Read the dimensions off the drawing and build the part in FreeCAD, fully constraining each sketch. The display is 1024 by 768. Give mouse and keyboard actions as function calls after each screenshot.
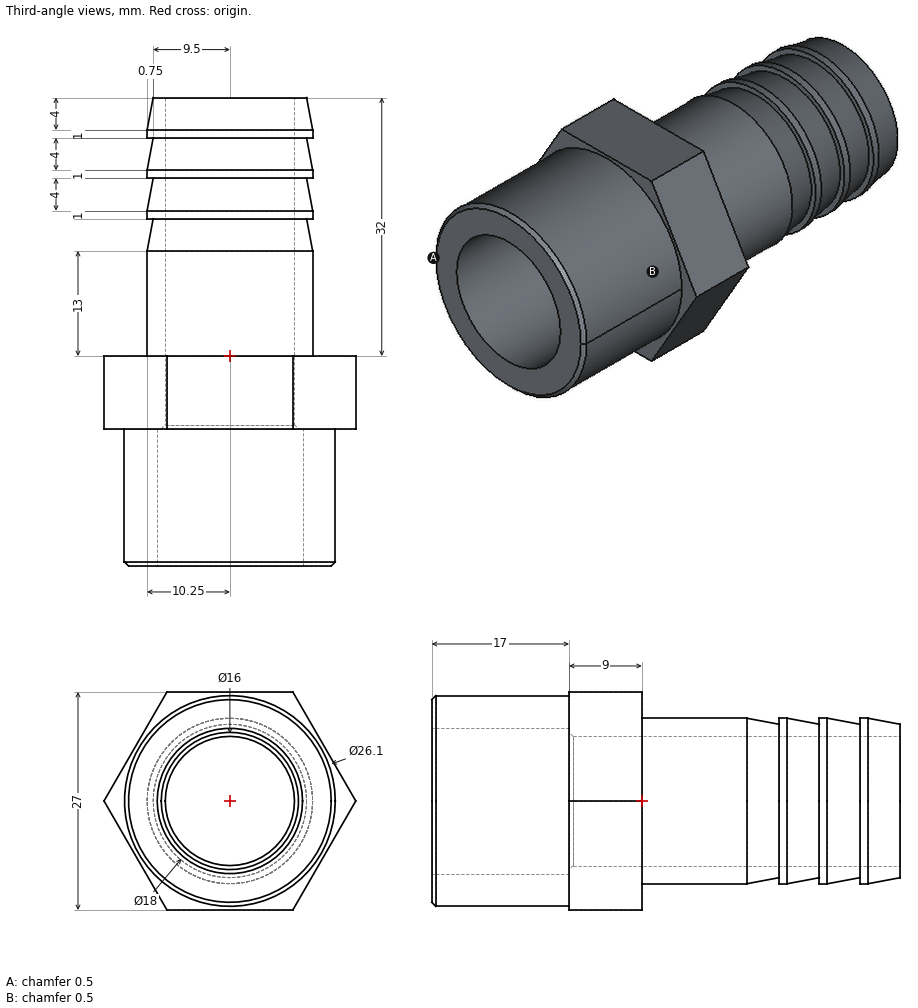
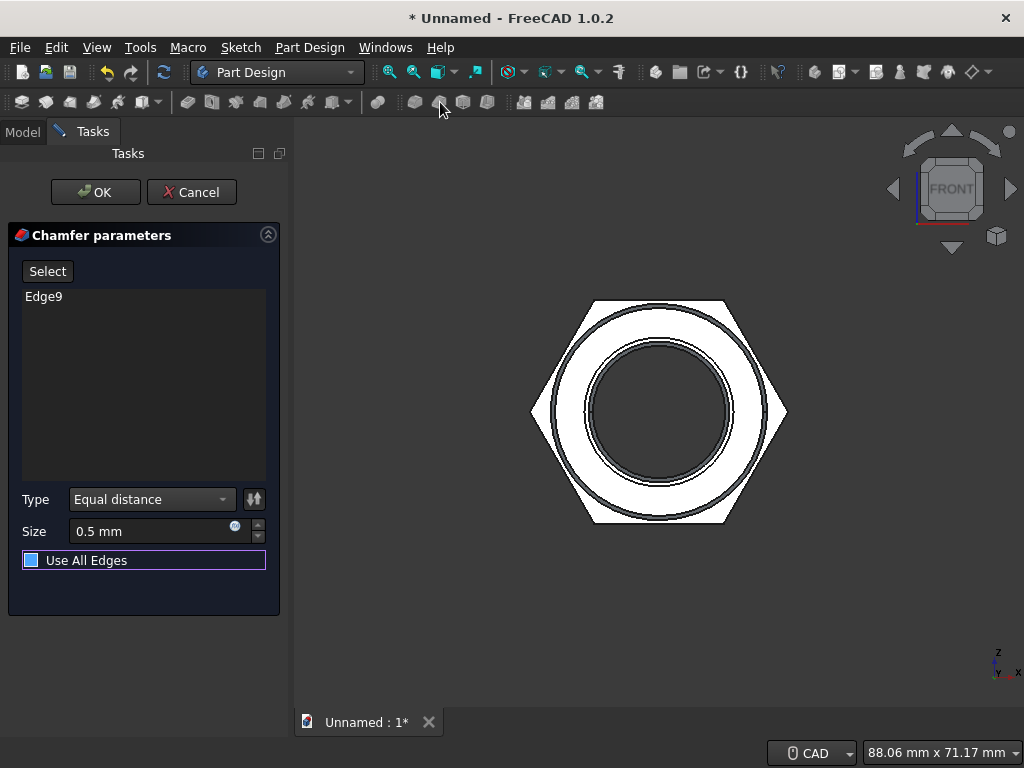
click(96, 192)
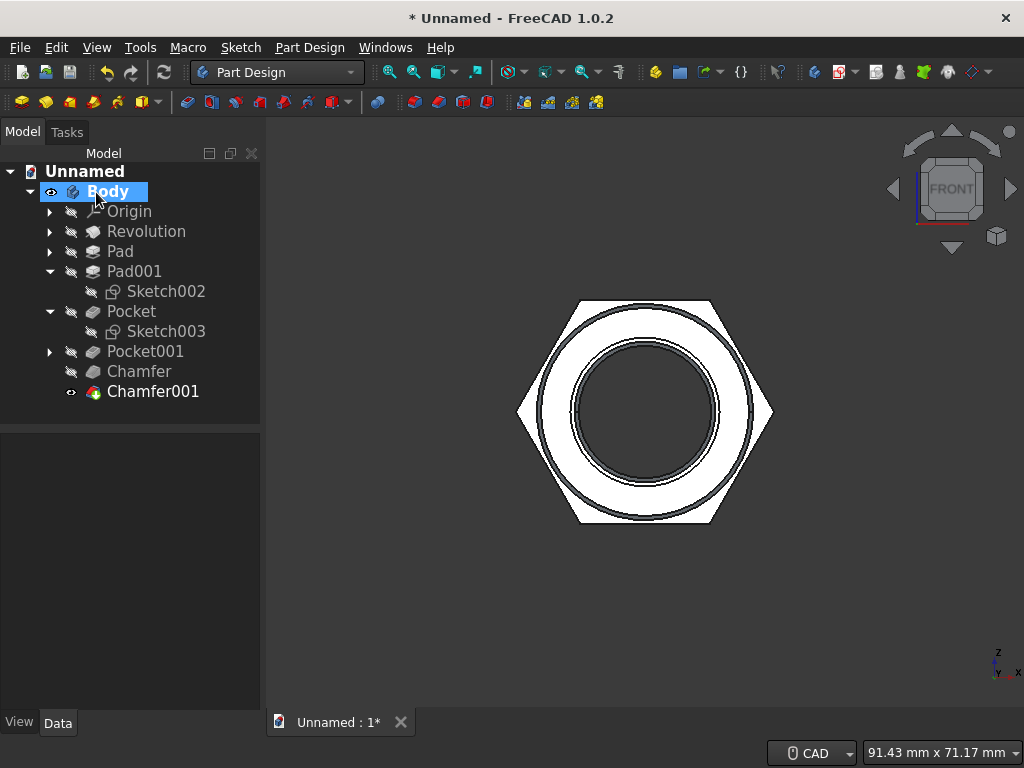
key(0)